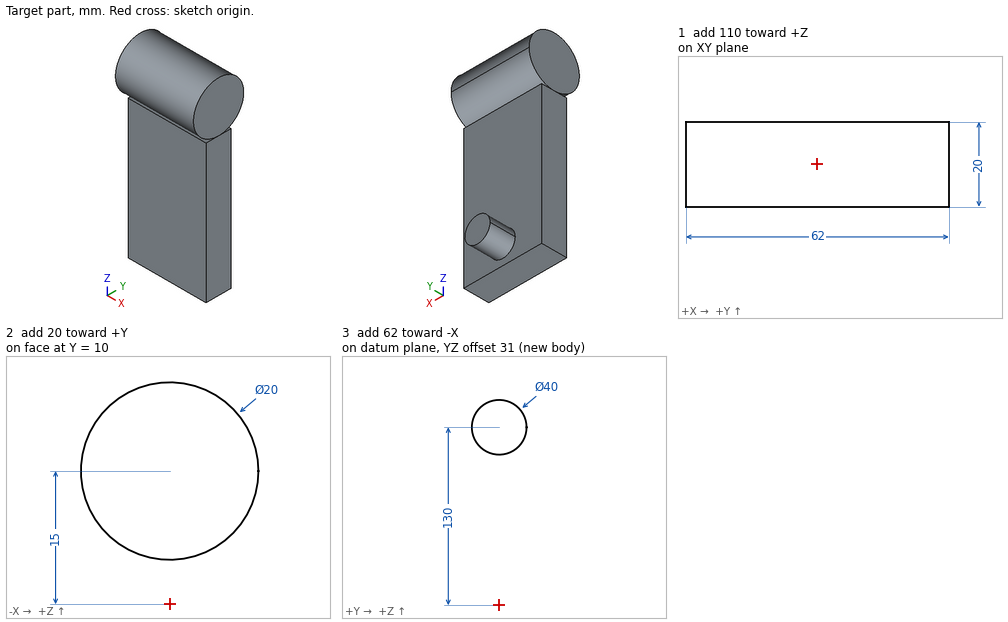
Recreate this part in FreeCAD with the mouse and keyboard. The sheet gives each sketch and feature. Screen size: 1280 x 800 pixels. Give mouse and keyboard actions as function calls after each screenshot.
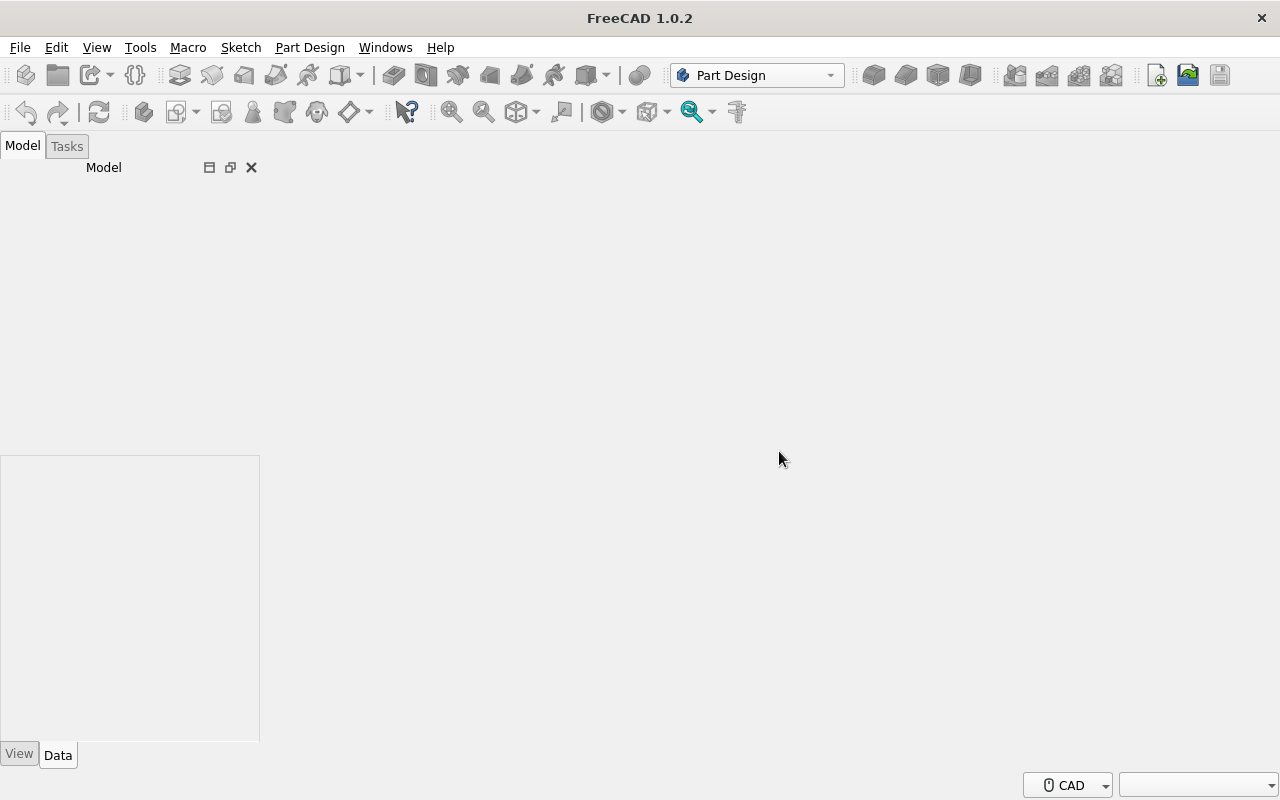
click(1156, 76)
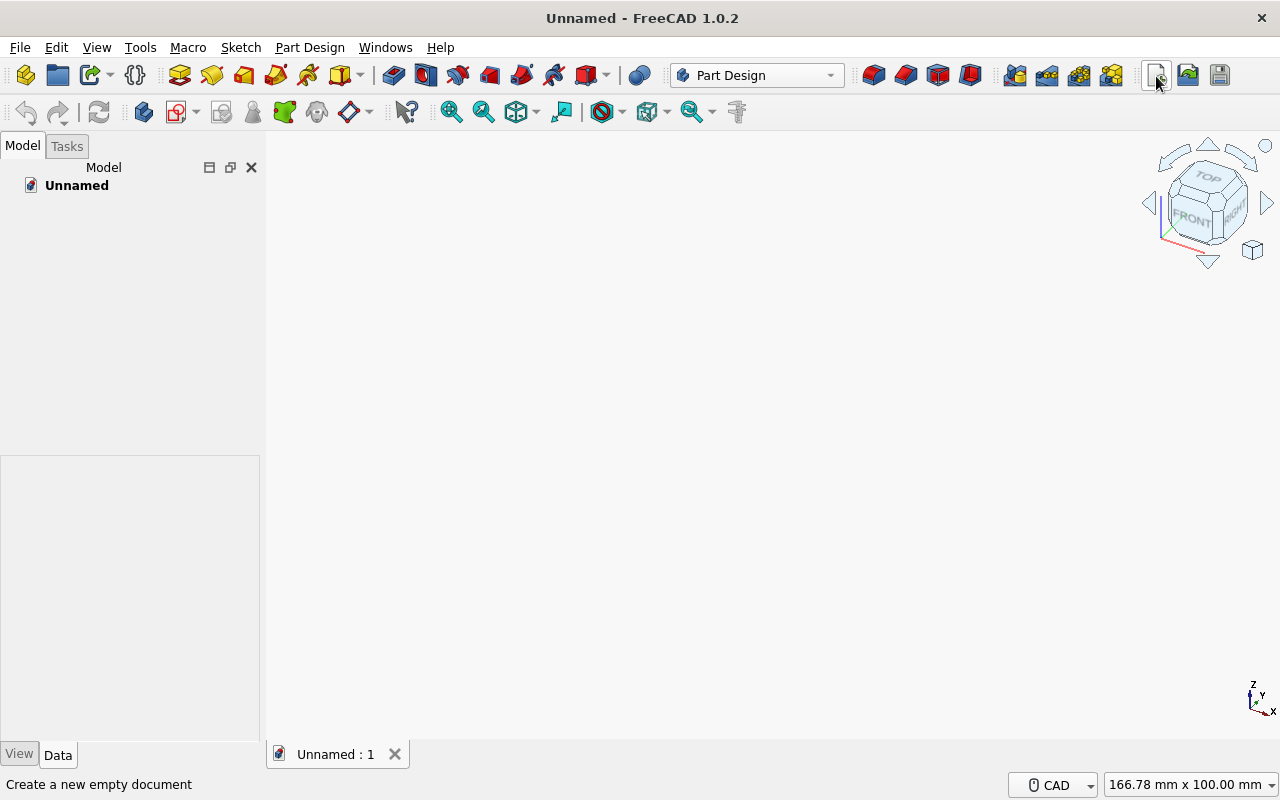
click(176, 112)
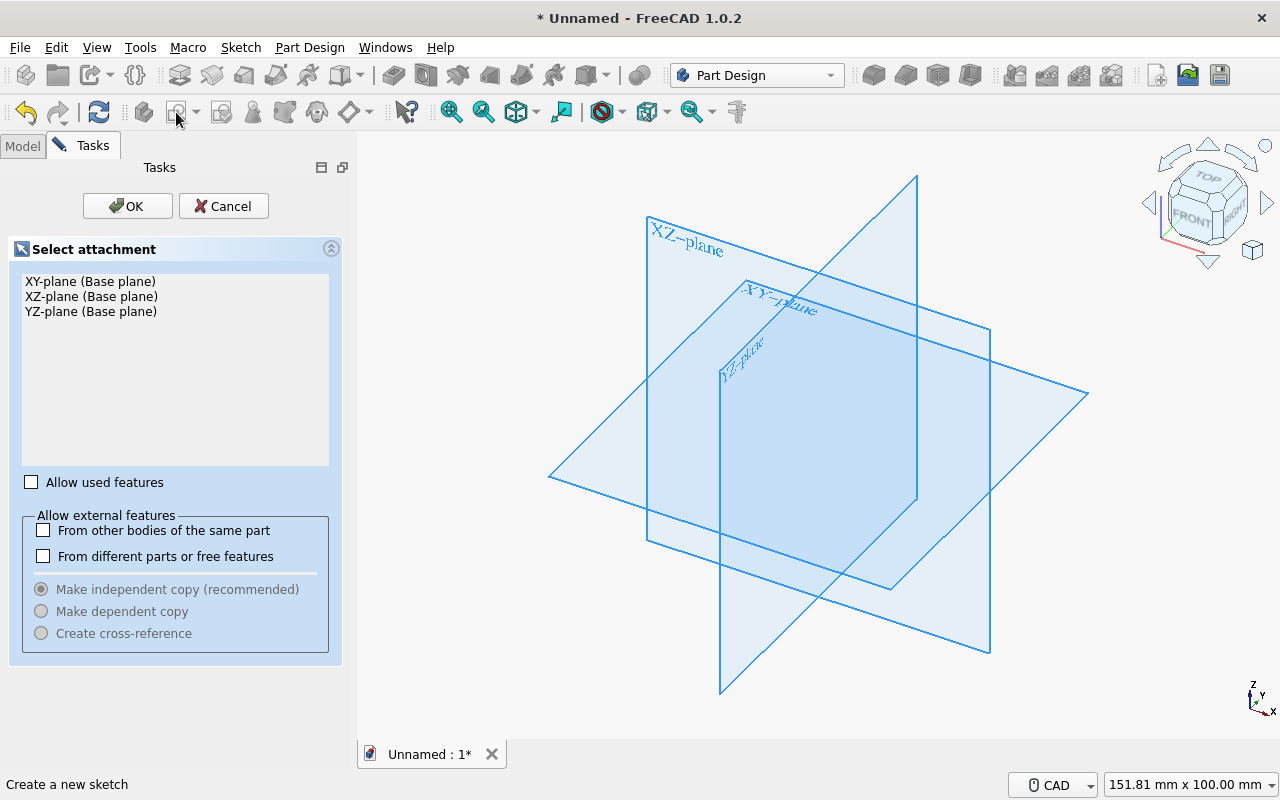
click(82, 282)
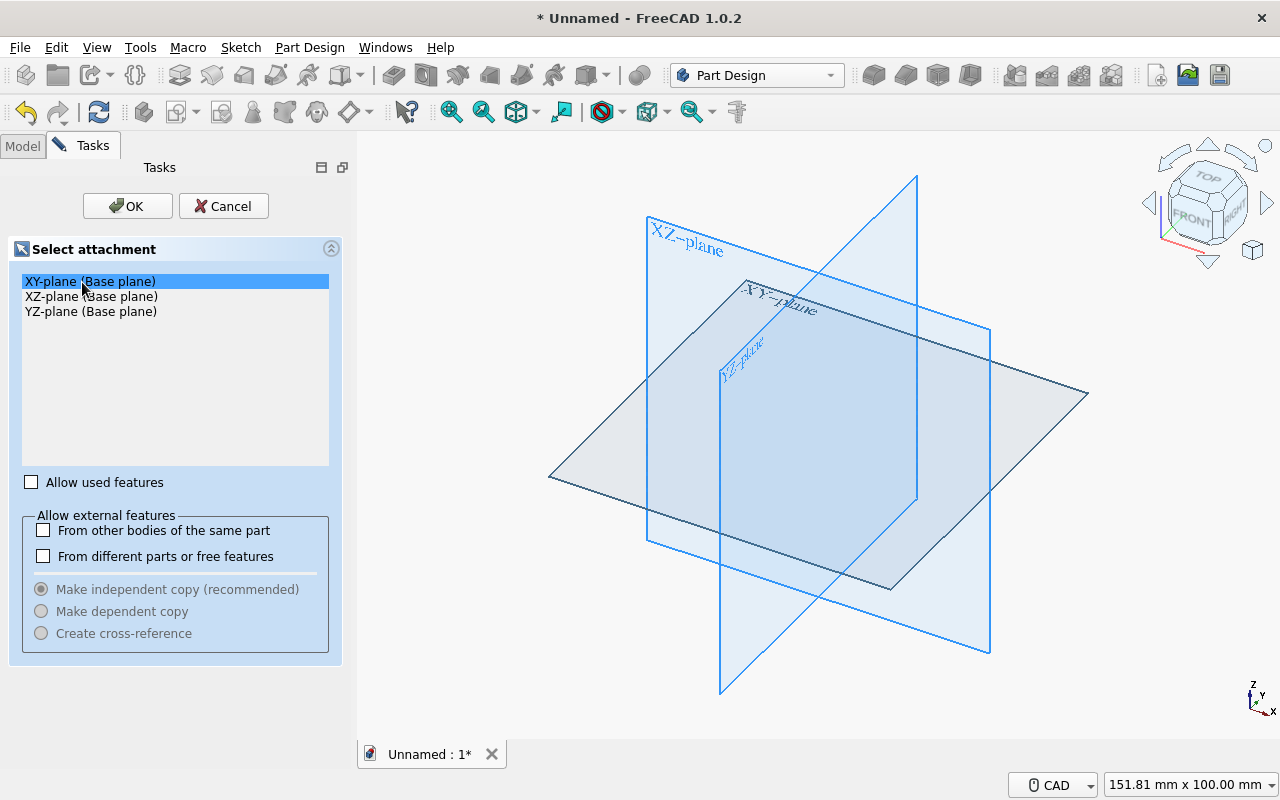
click(128, 206)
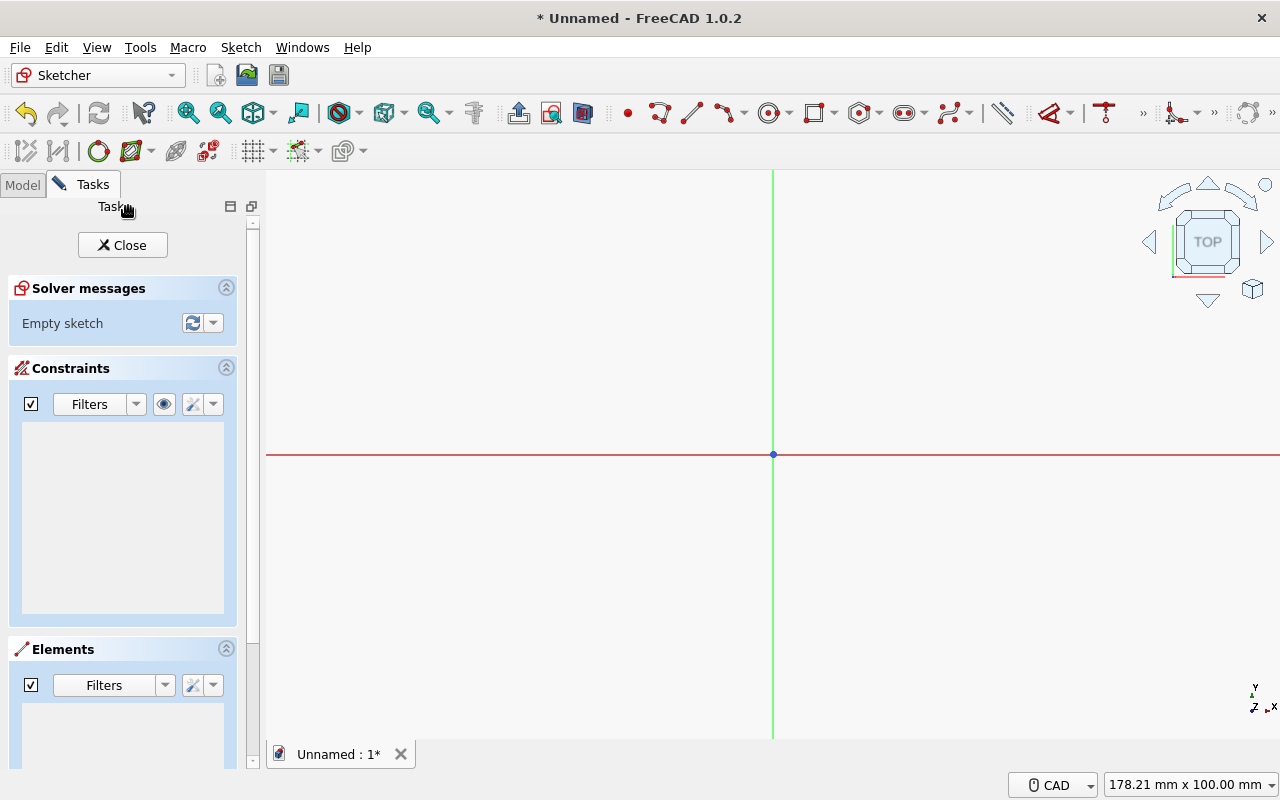
scroll(912, 455, up, 2)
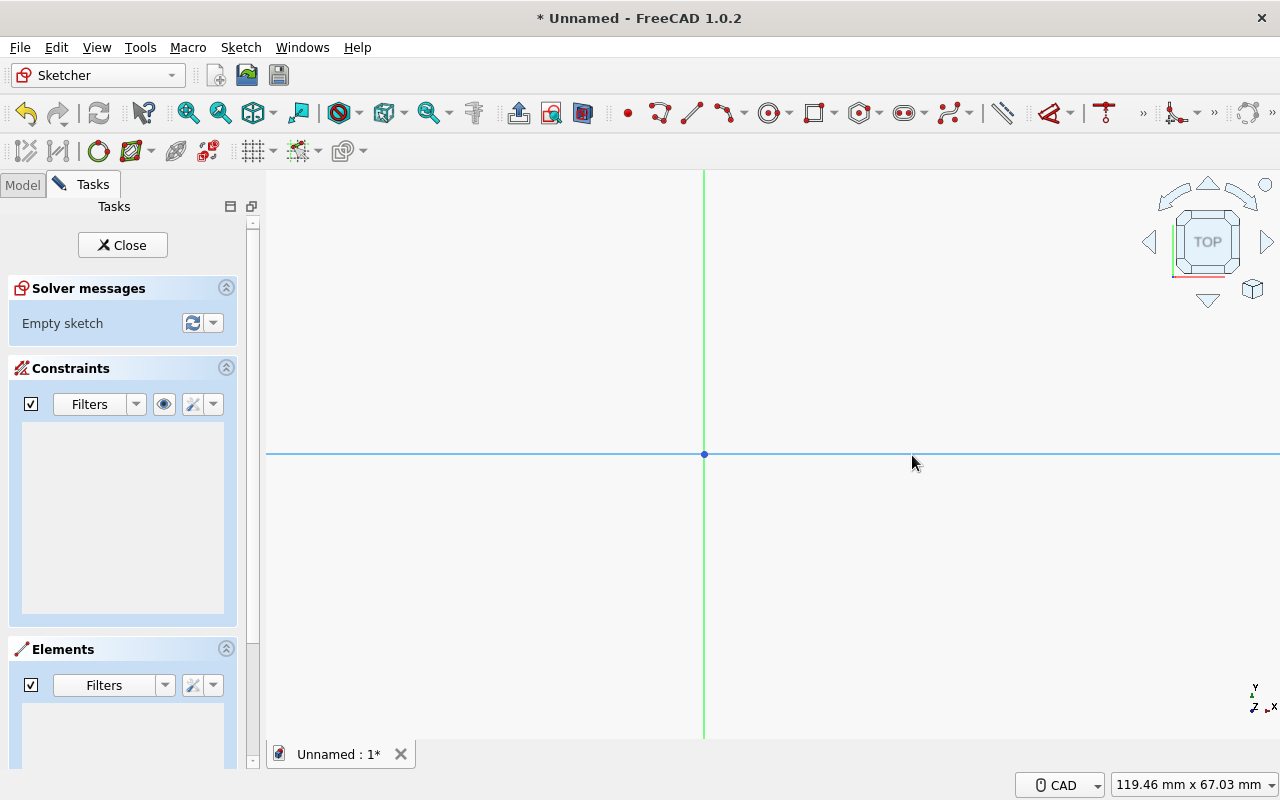
key(g)
key(v)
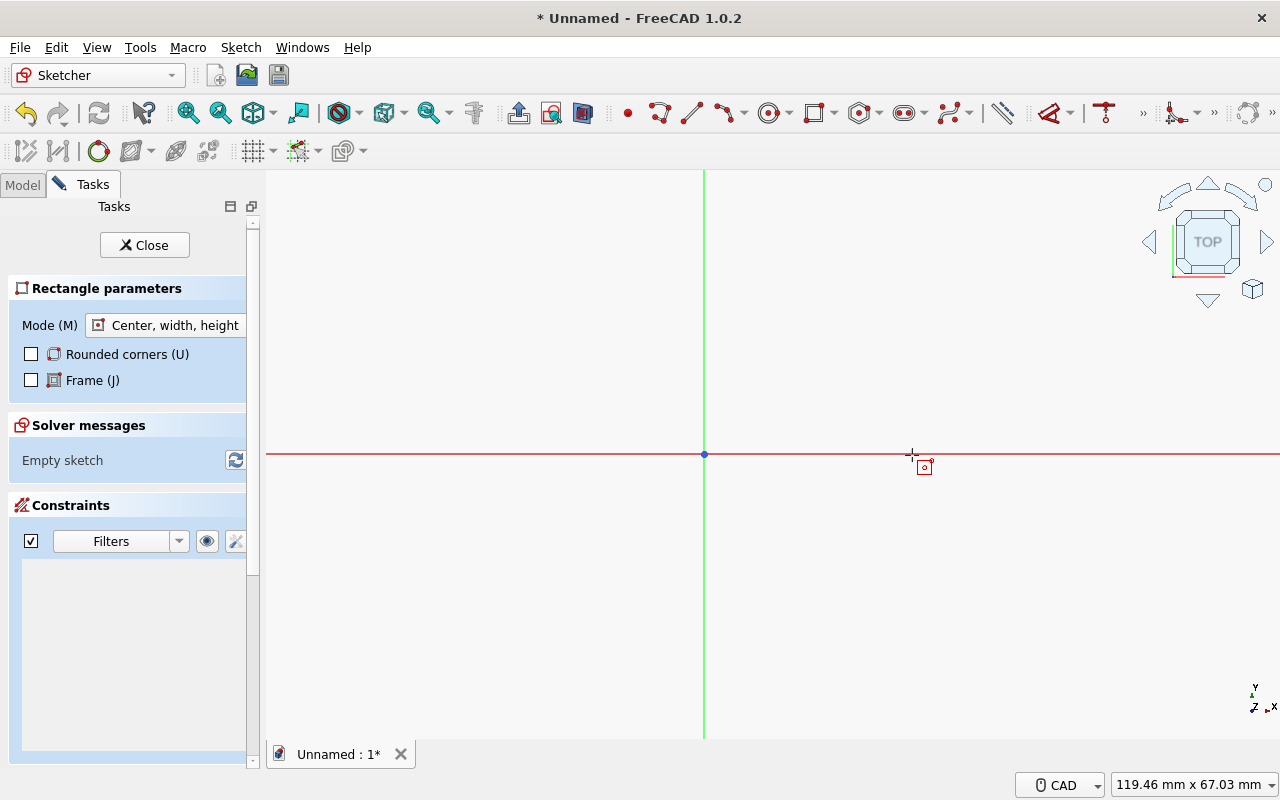
click(704, 454)
move(967, 369)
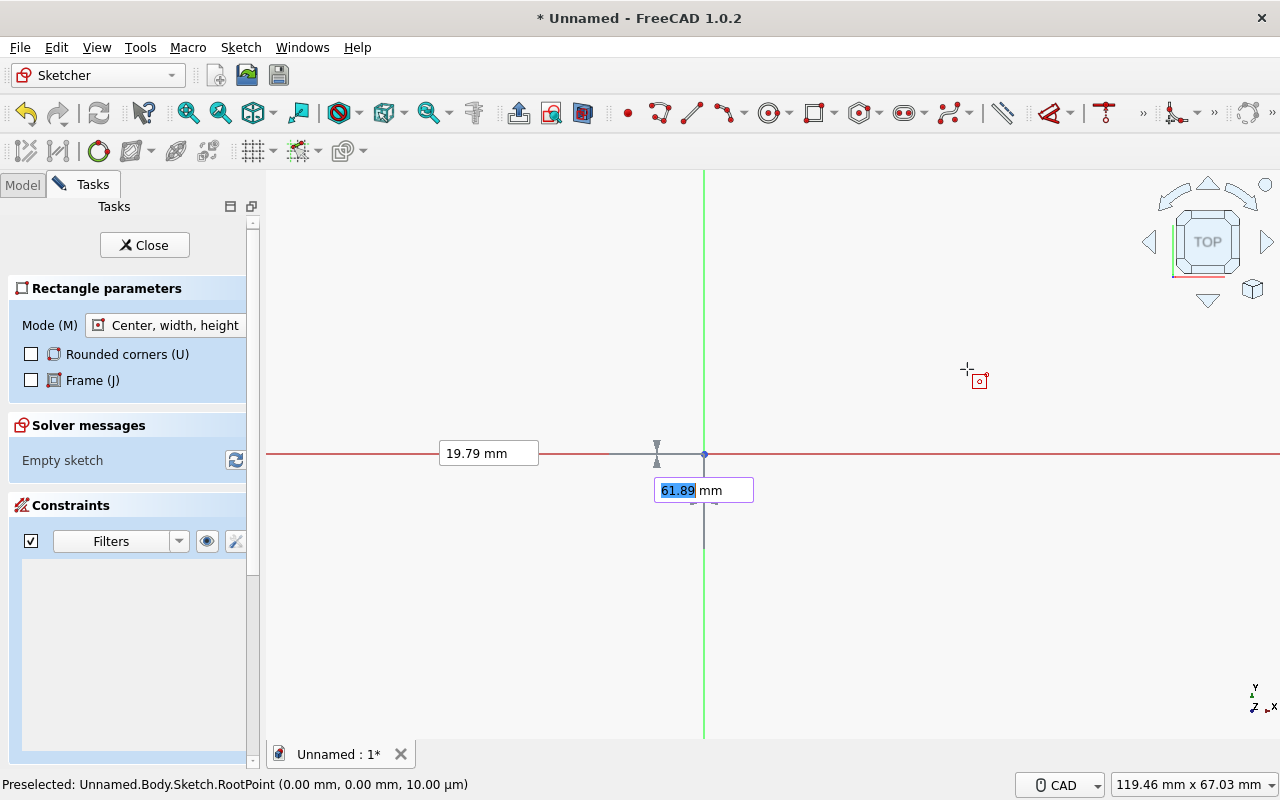
text(62)
key(Tab)
text(20)
key(Return)
key(Escape)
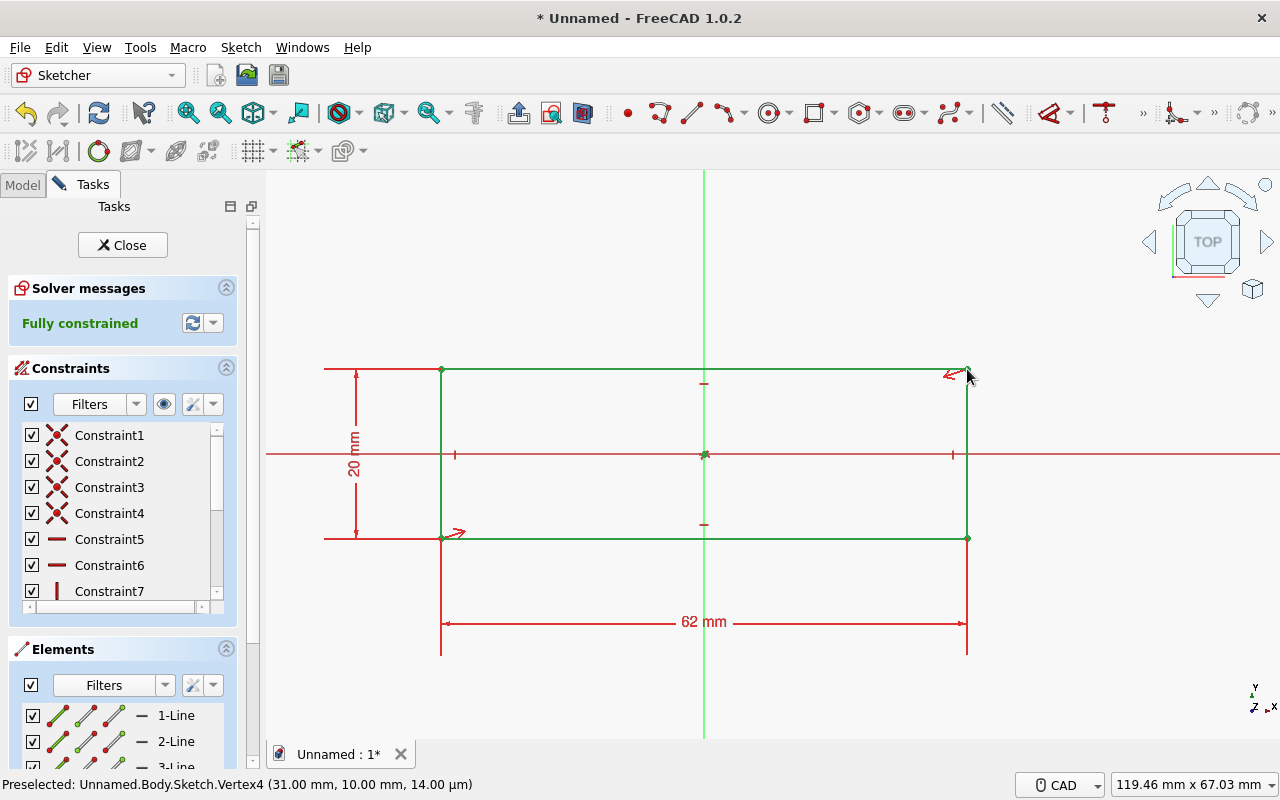
click(123, 245)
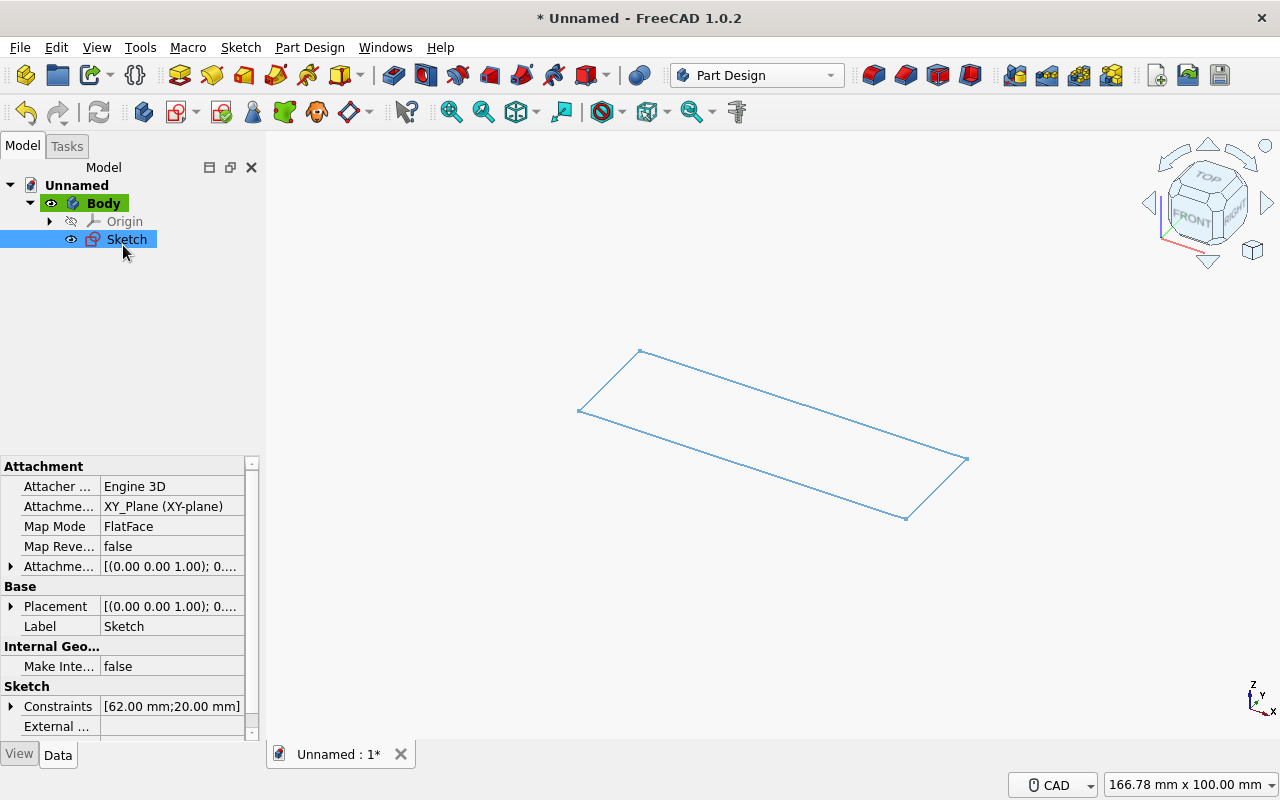
click(180, 76)